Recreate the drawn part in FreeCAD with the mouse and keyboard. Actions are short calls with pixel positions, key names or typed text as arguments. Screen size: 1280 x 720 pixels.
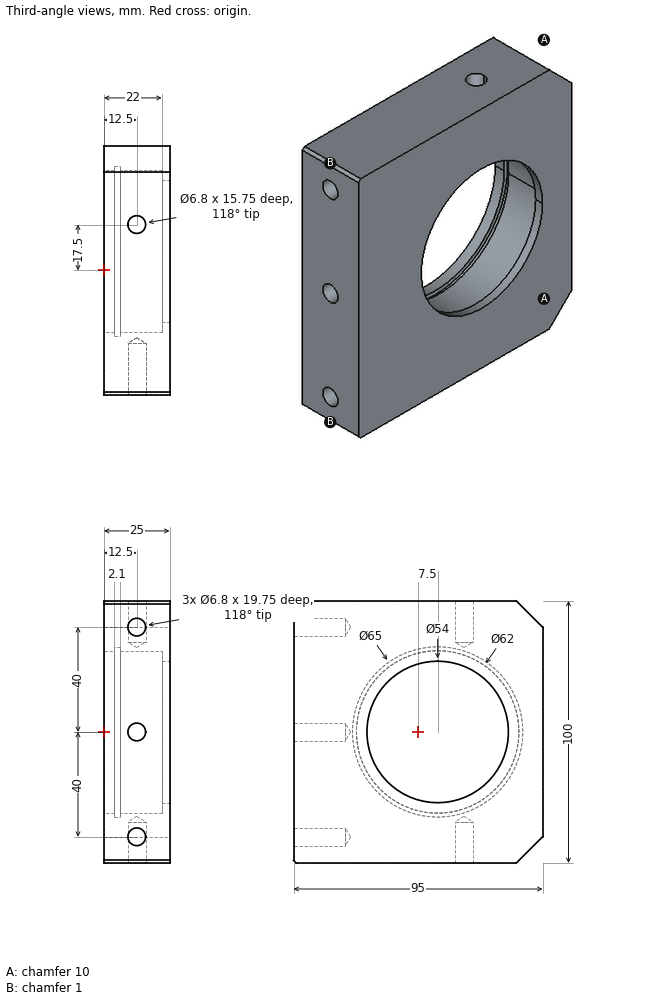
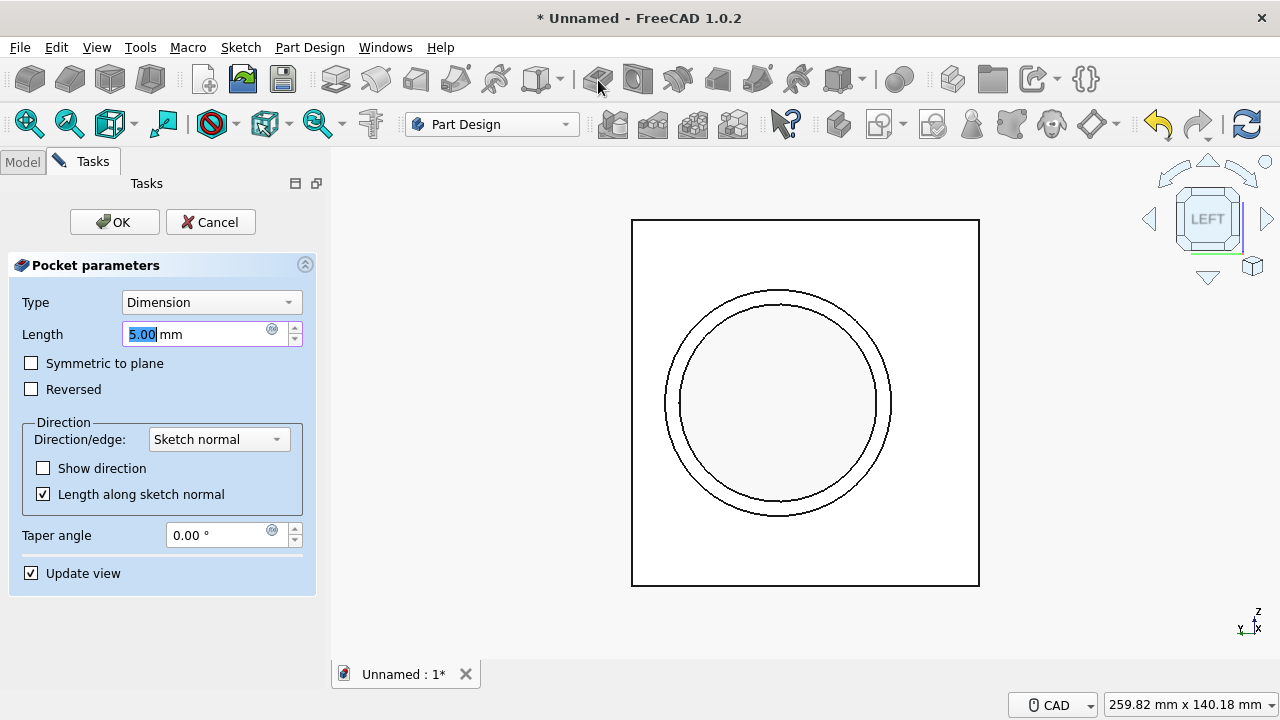
click(212, 302)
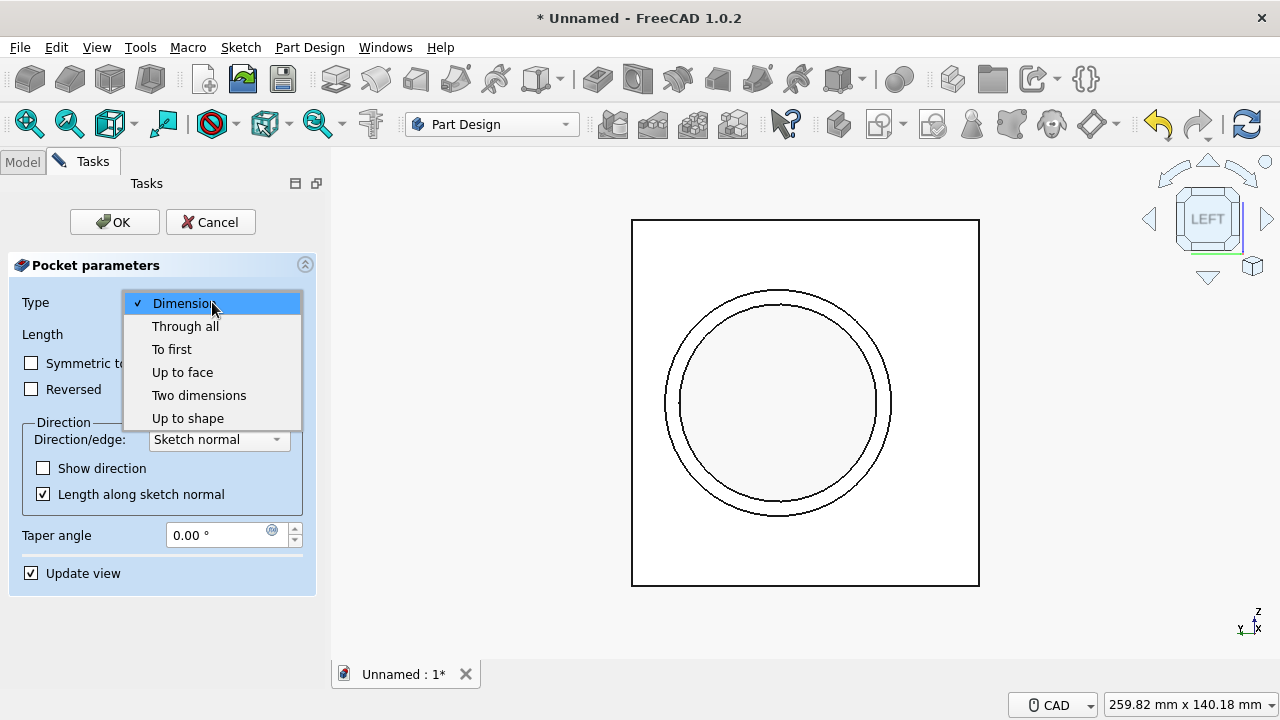
click(212, 326)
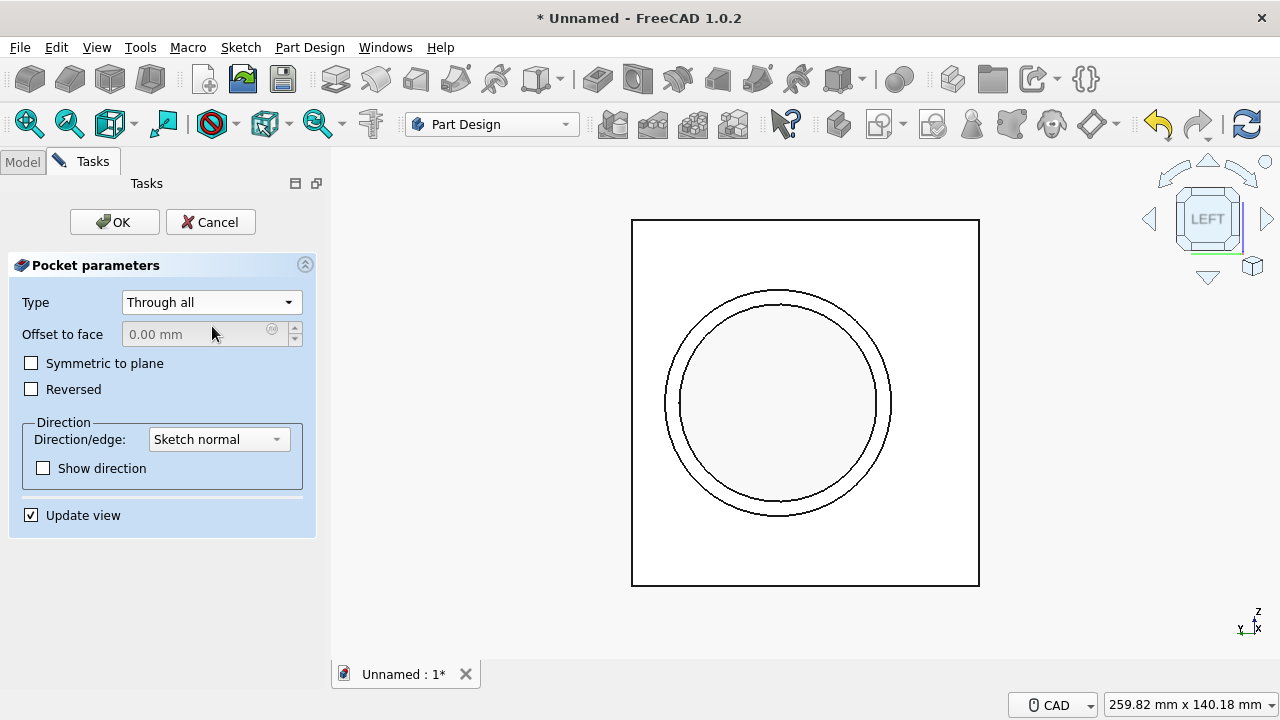
click(115, 222)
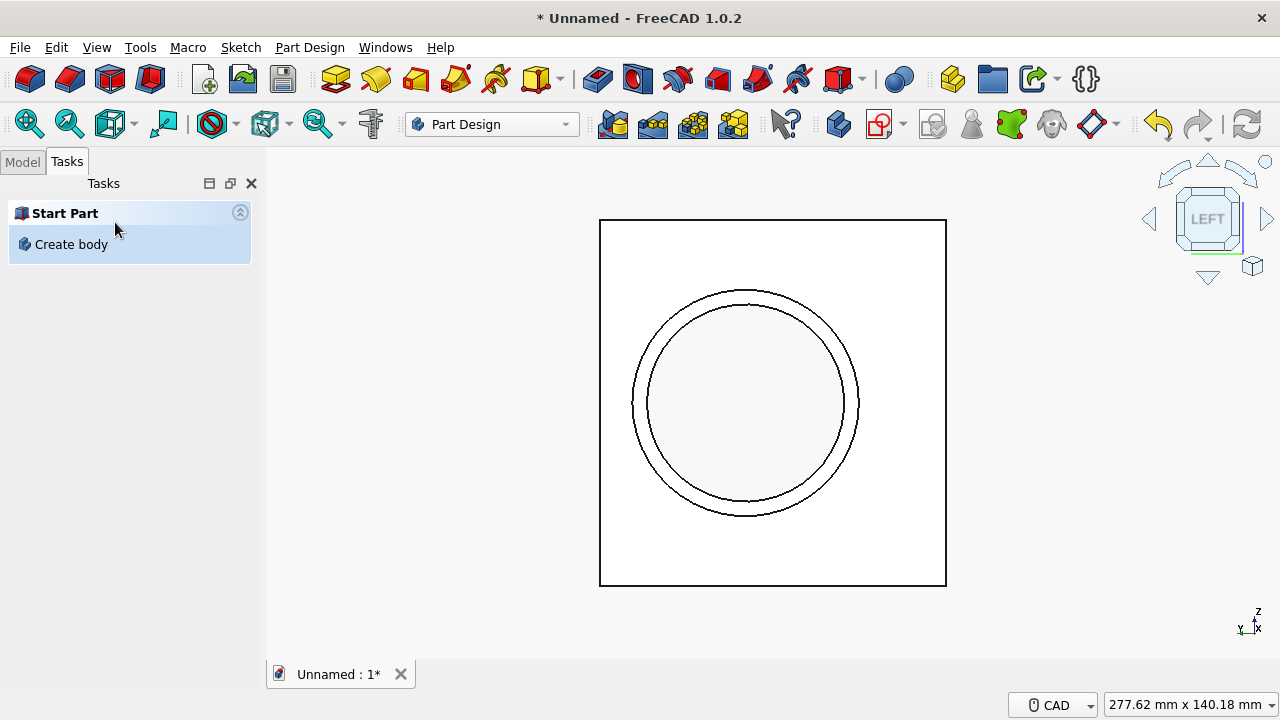
click(23, 161)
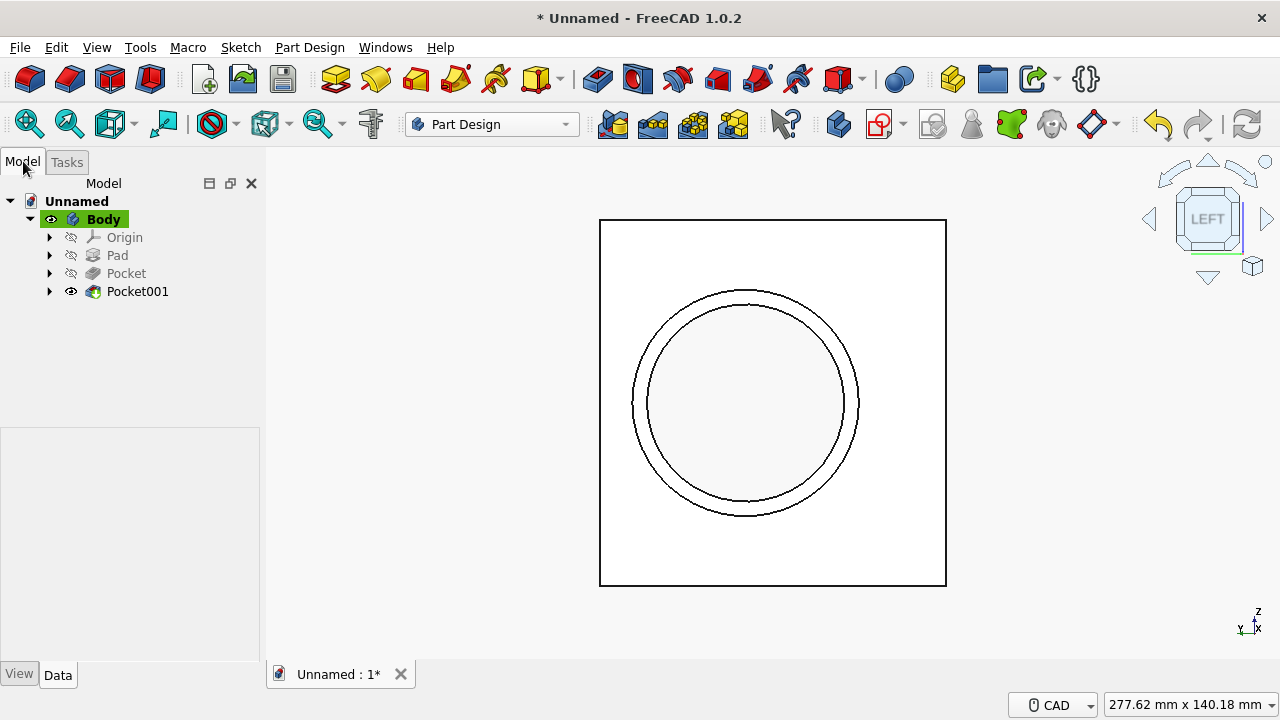
click(50, 237)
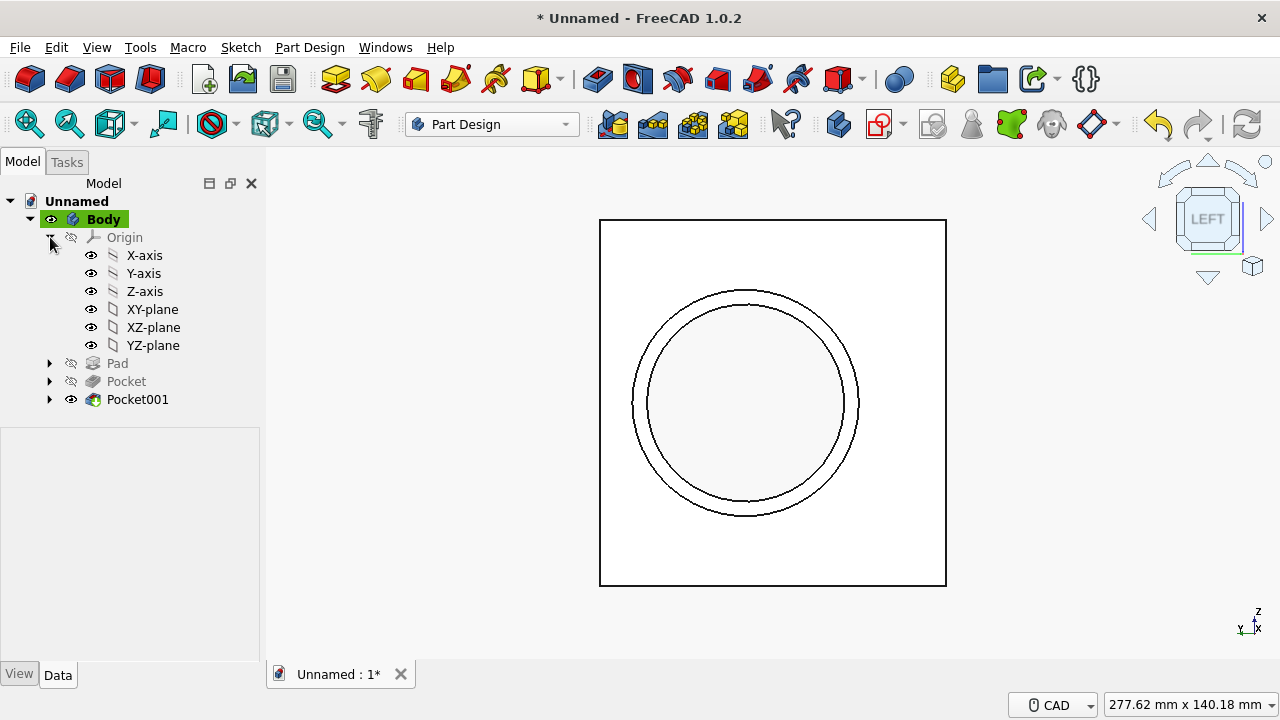
click(136, 345)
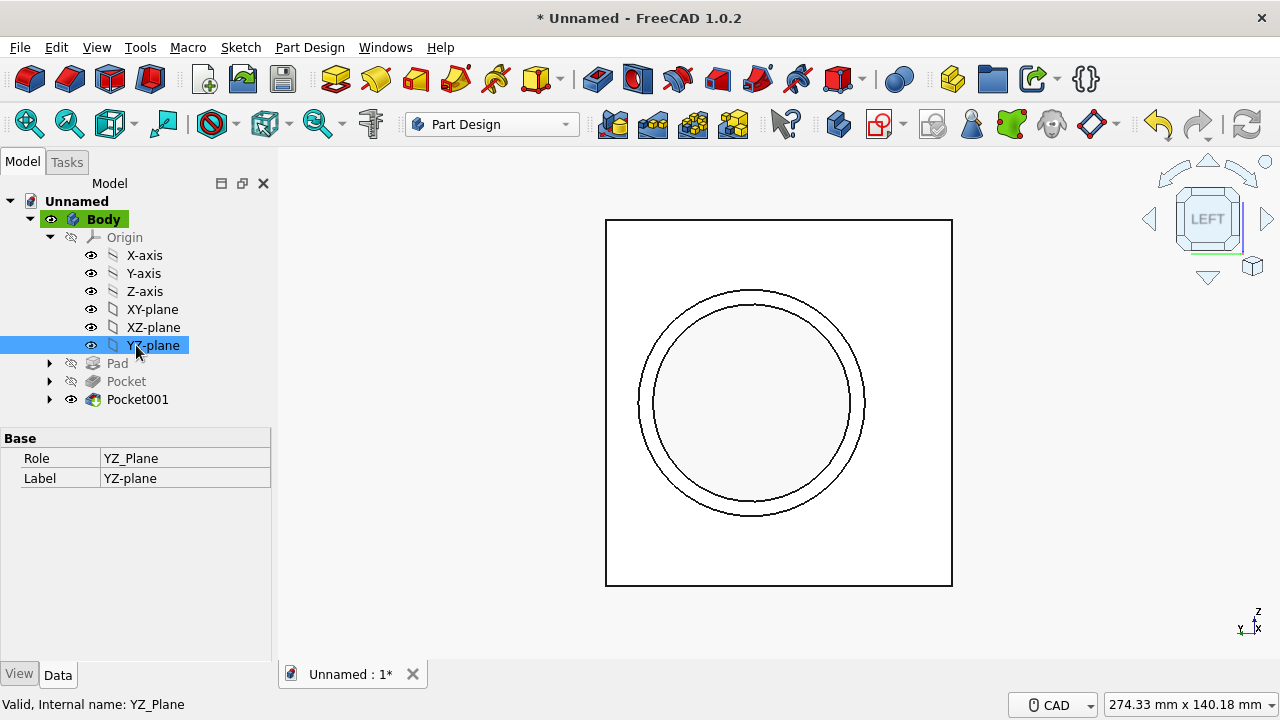
click(1092, 124)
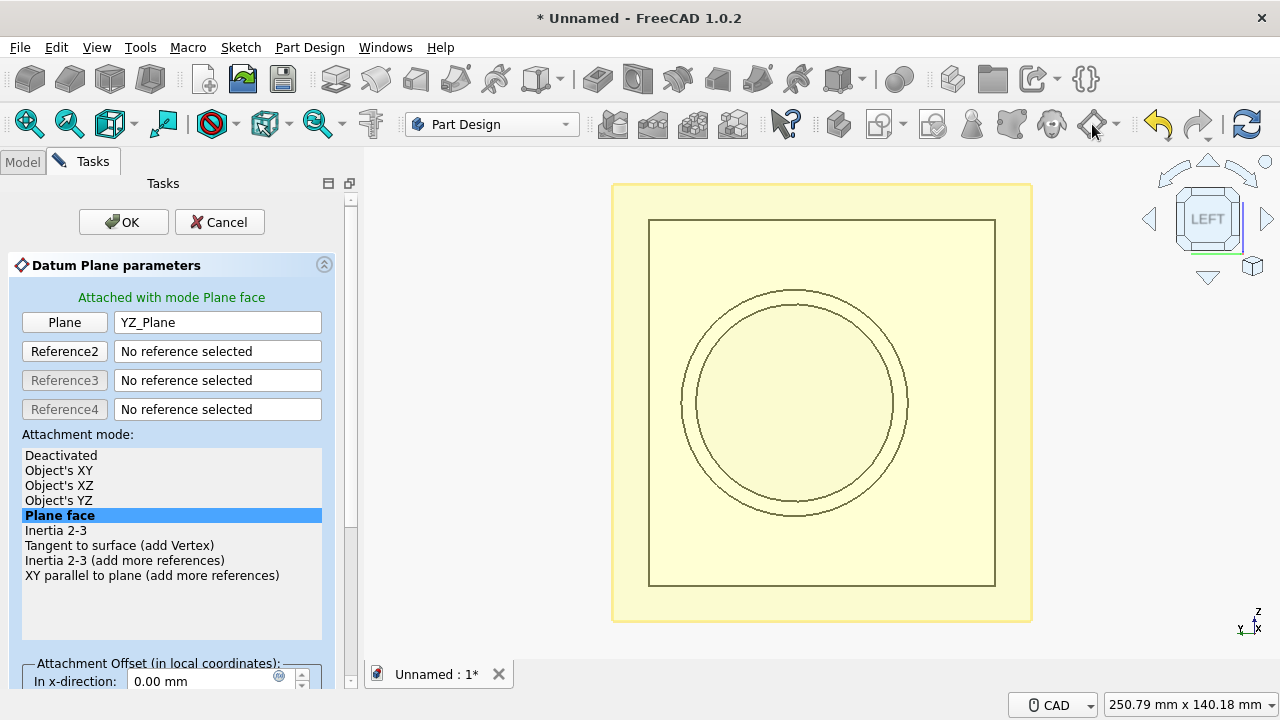
scroll(351, 440, down, 3)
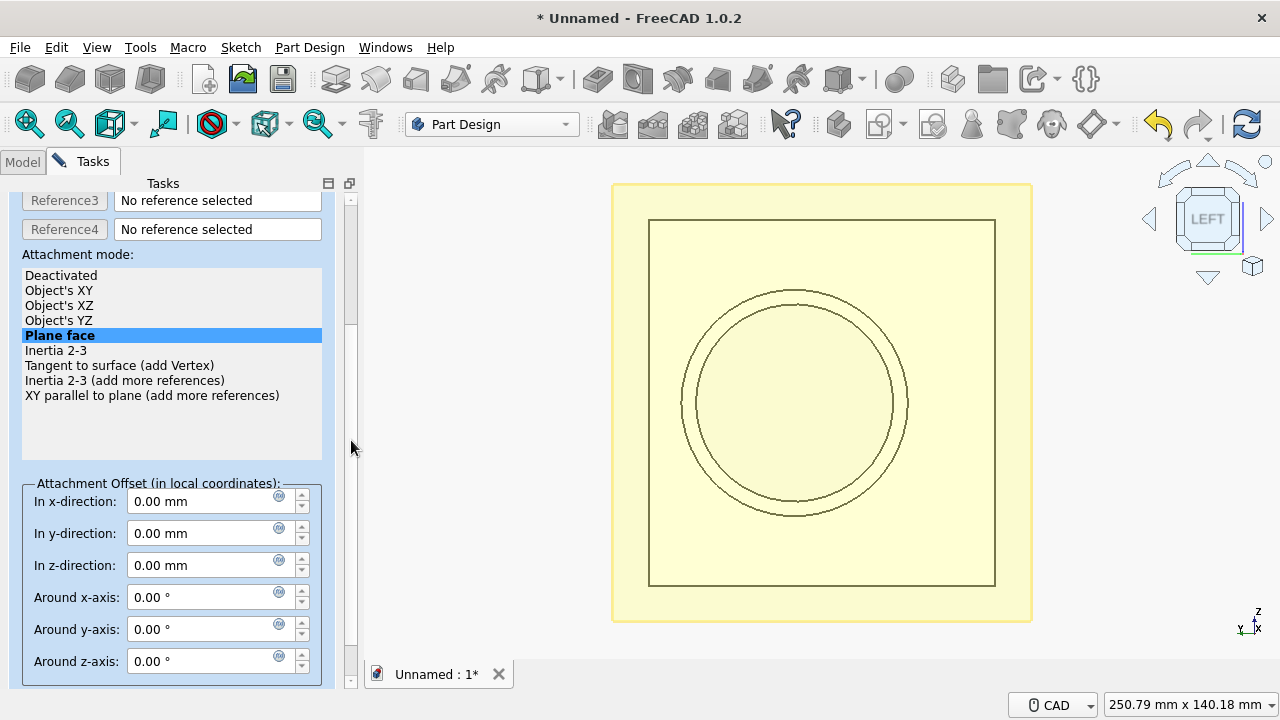
triple_click(210, 565)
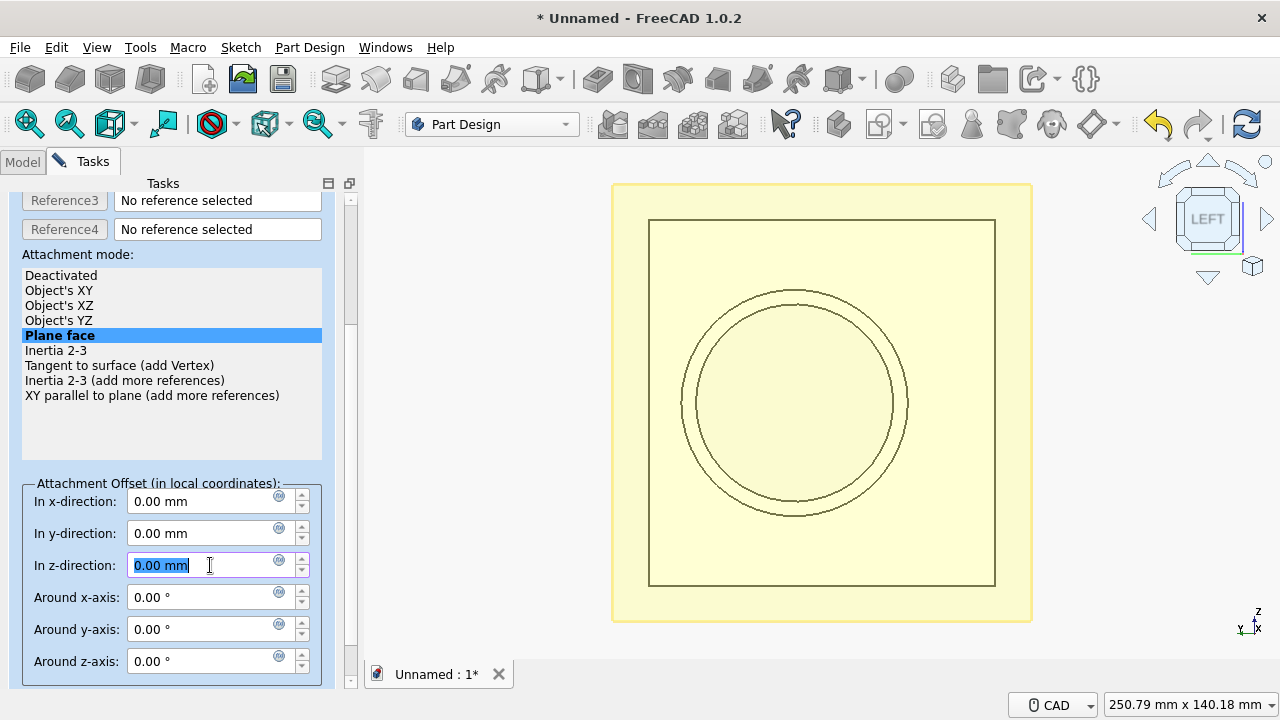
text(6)
key(Tab)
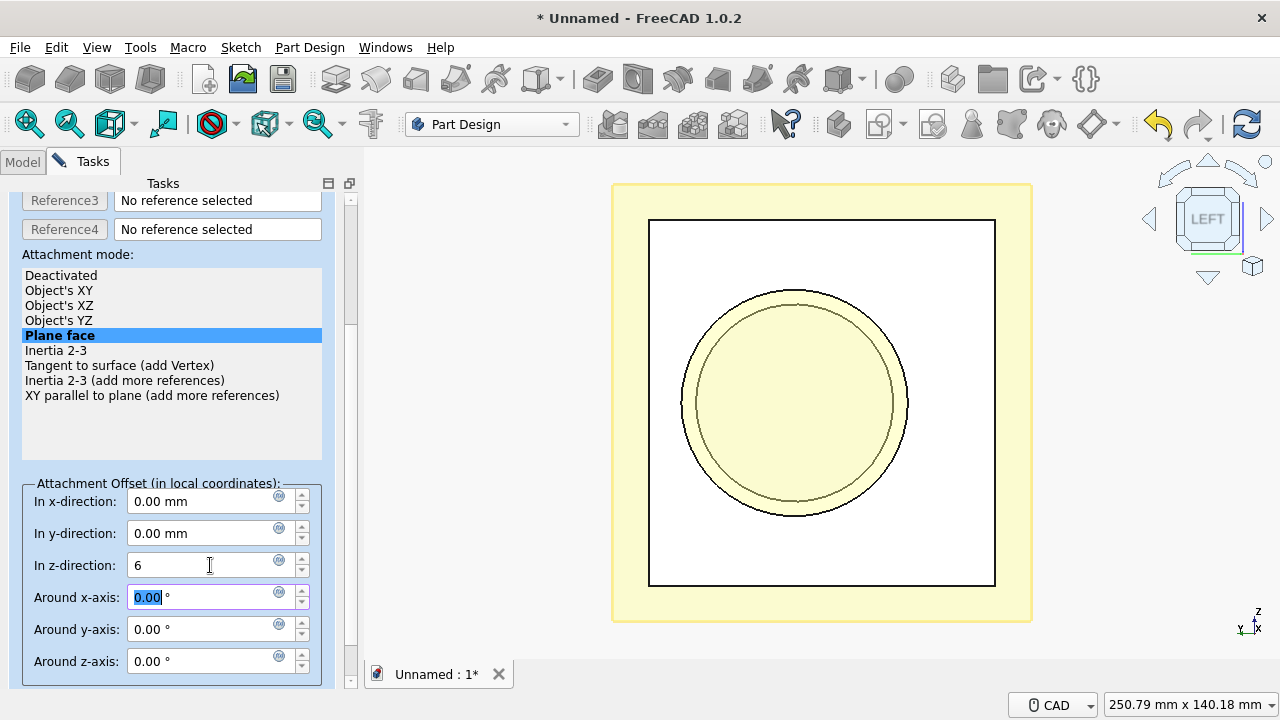
scroll(351, 440, up, 4)